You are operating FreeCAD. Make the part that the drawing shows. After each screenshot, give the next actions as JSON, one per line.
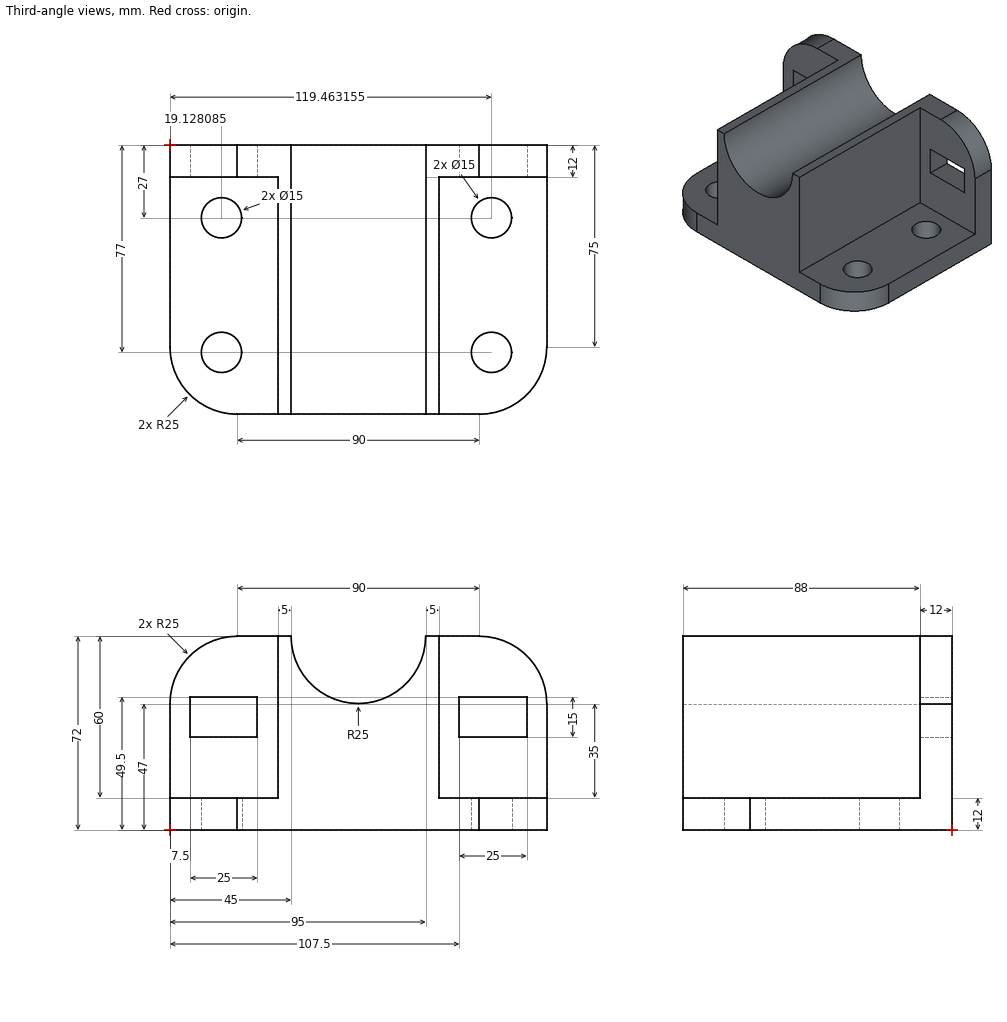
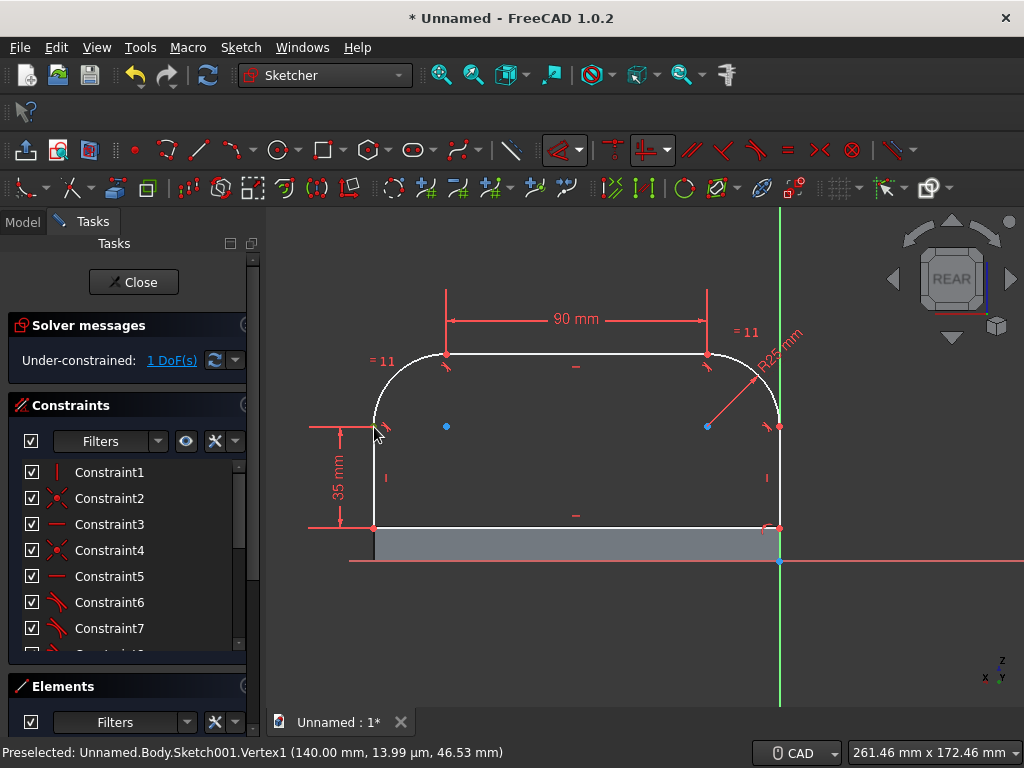
{"action": "left_click", "coordinate": [582, 150]}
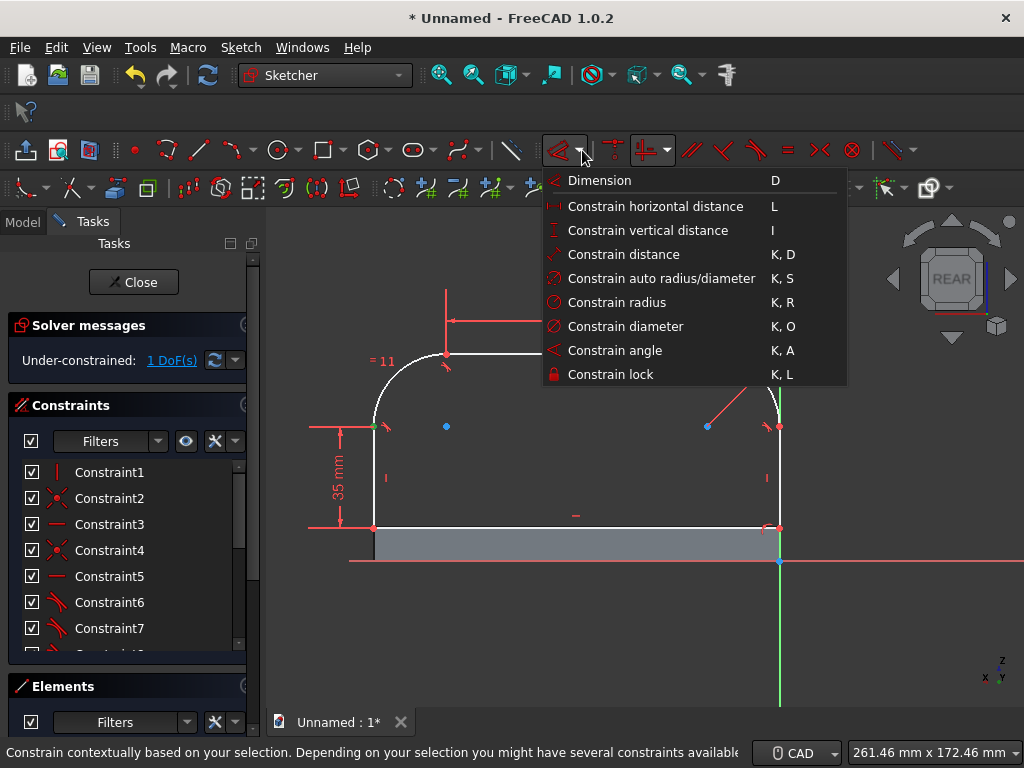
{"action": "left_click", "coordinate": [695, 230]}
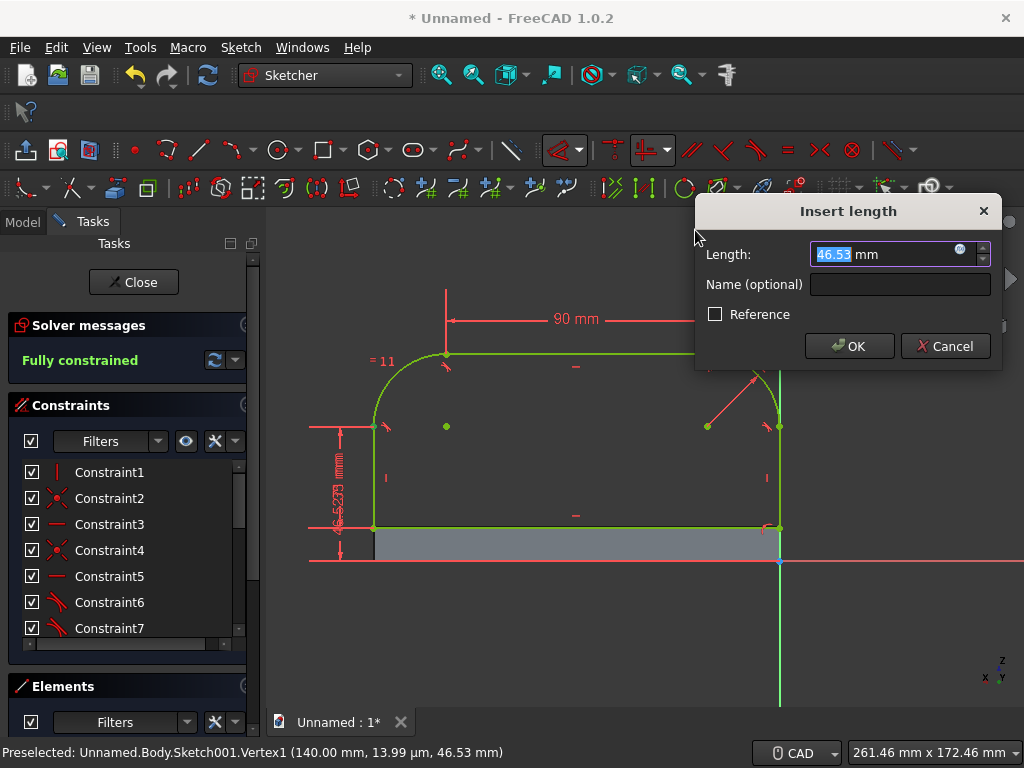
{"action": "type", "text": "47"}
{"action": "key", "text": "Return"}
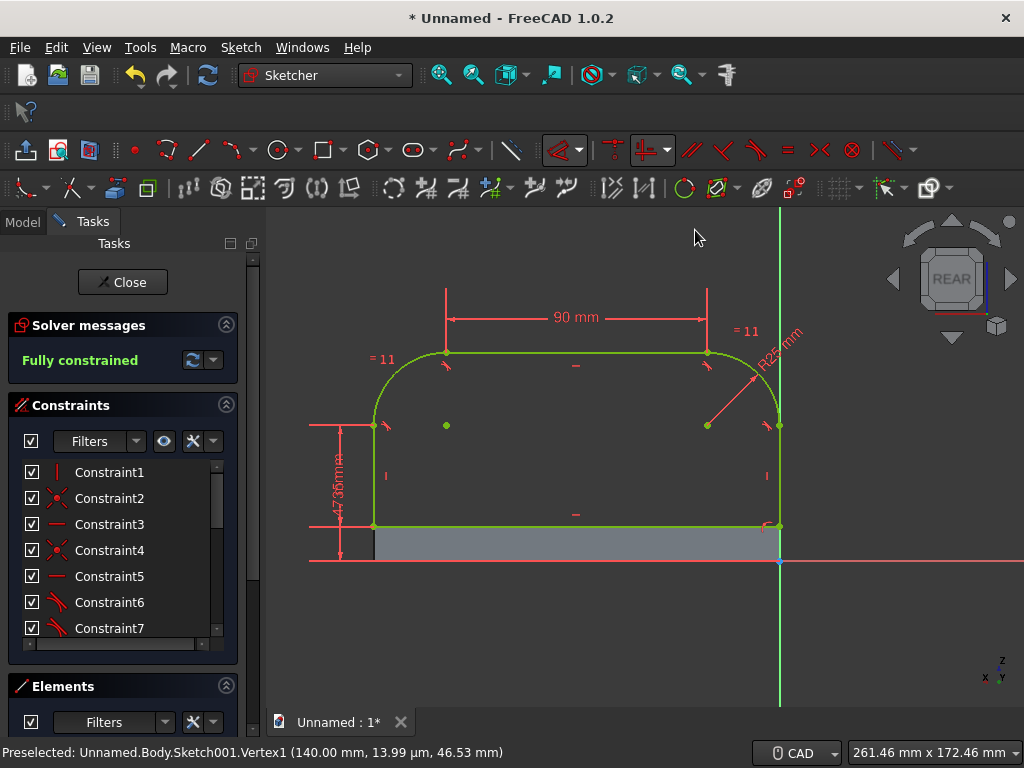
{"action": "left_click", "coordinate": [123, 282]}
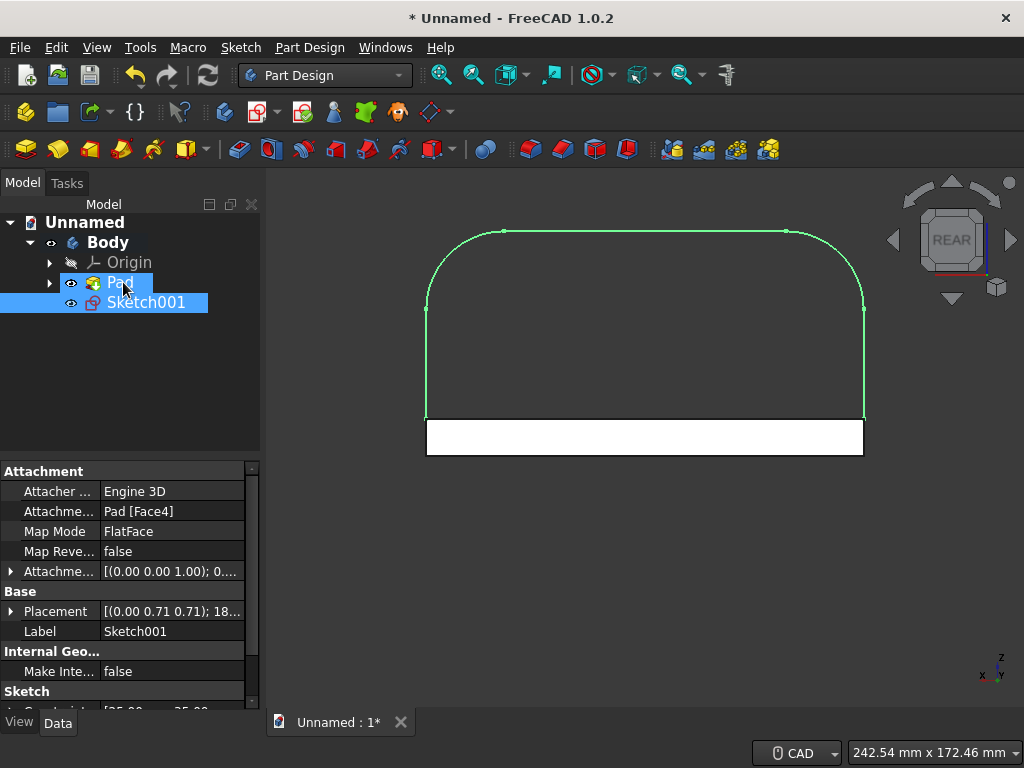
{"action": "left_click", "coordinate": [26, 150]}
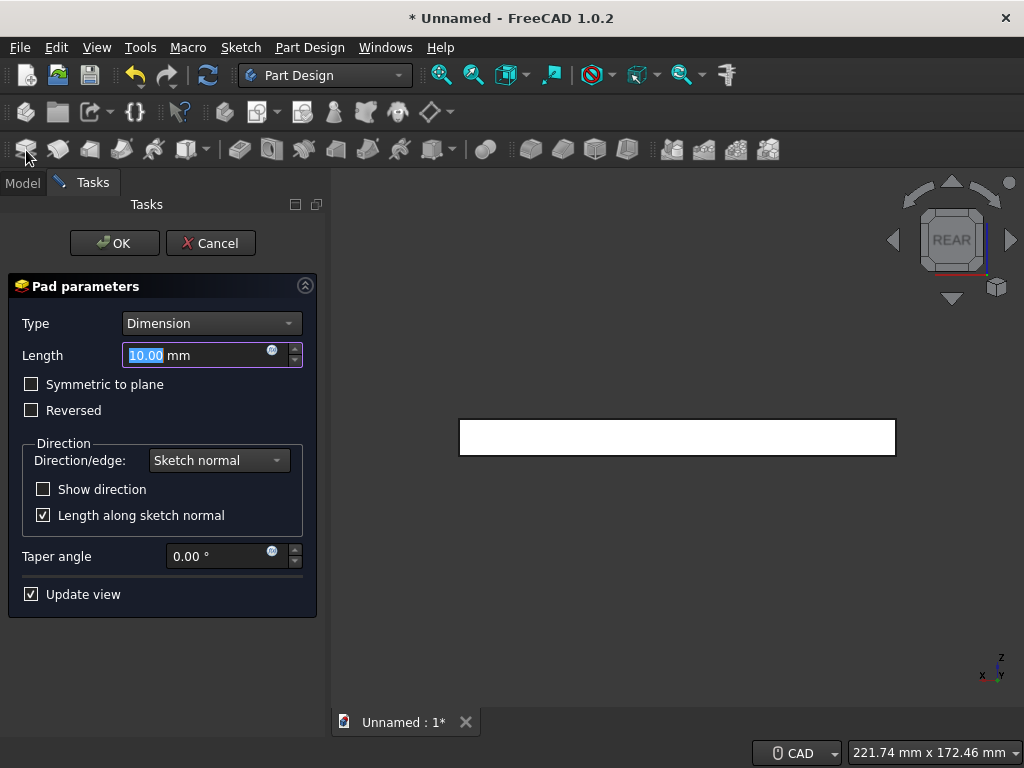
{"action": "type", "text": "12"}
{"action": "key", "text": "Tab"}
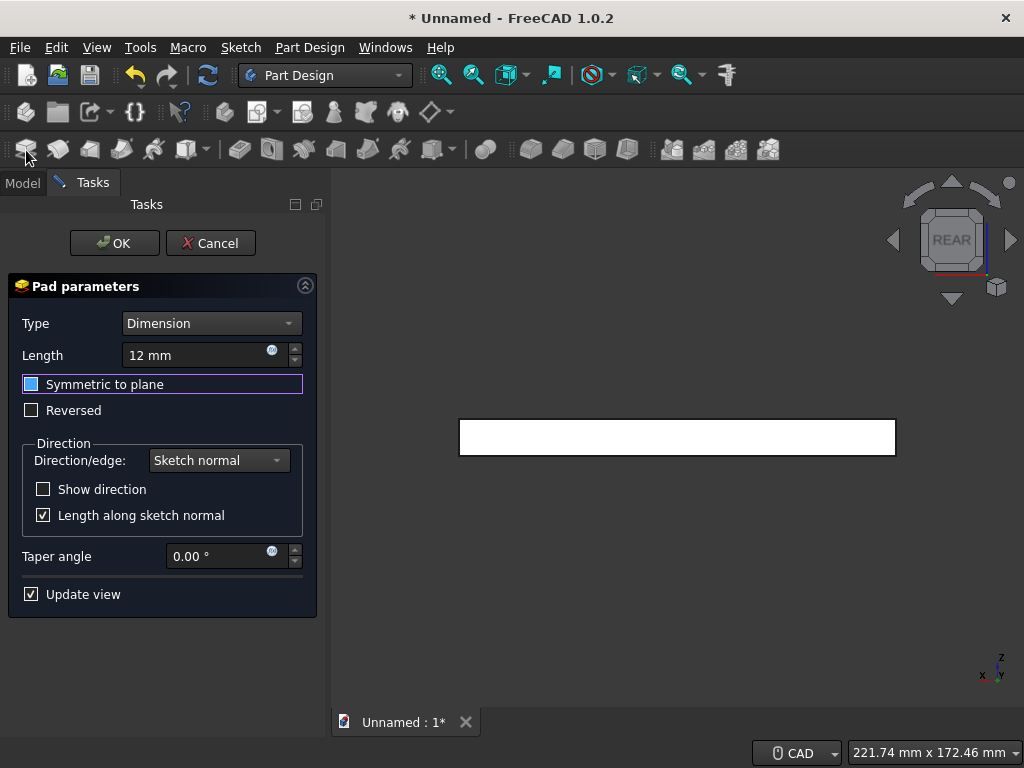
{"action": "left_click", "coordinate": [30, 410]}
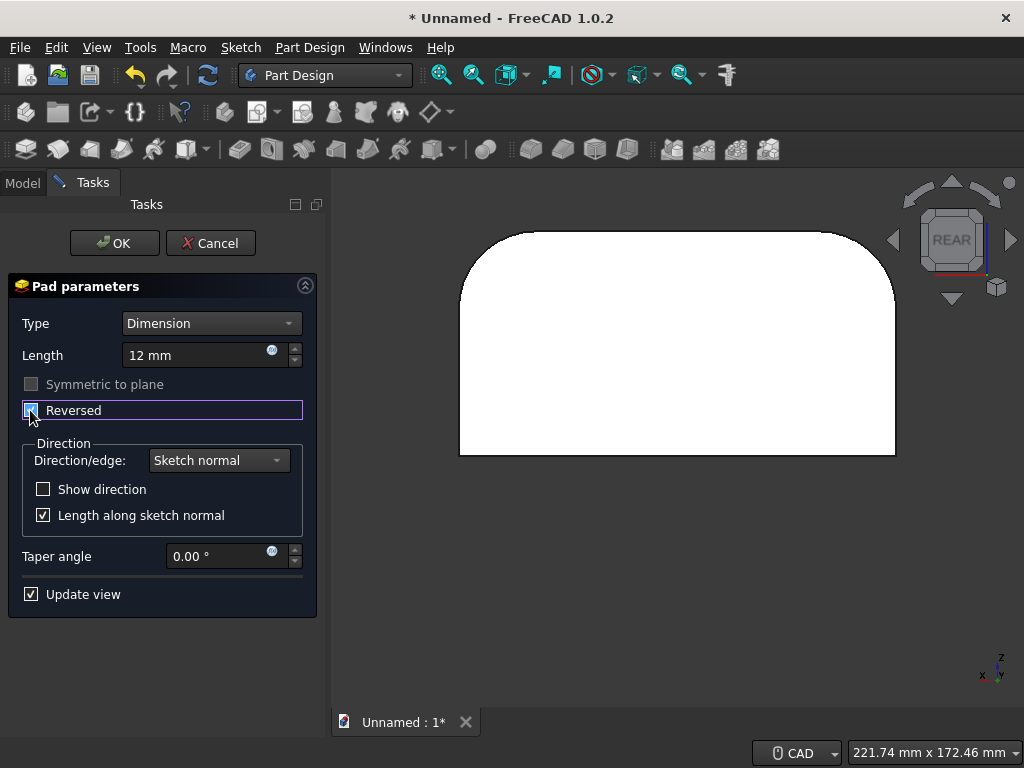
{"action": "left_click", "coordinate": [115, 243]}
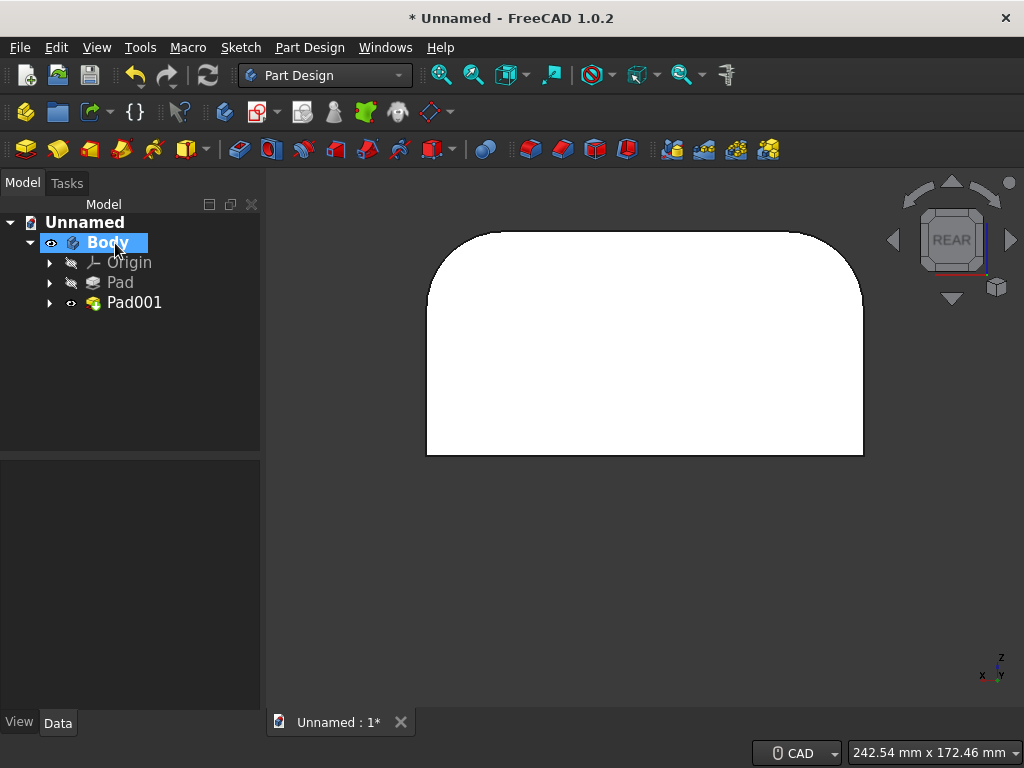
{"action": "key", "text": "0"}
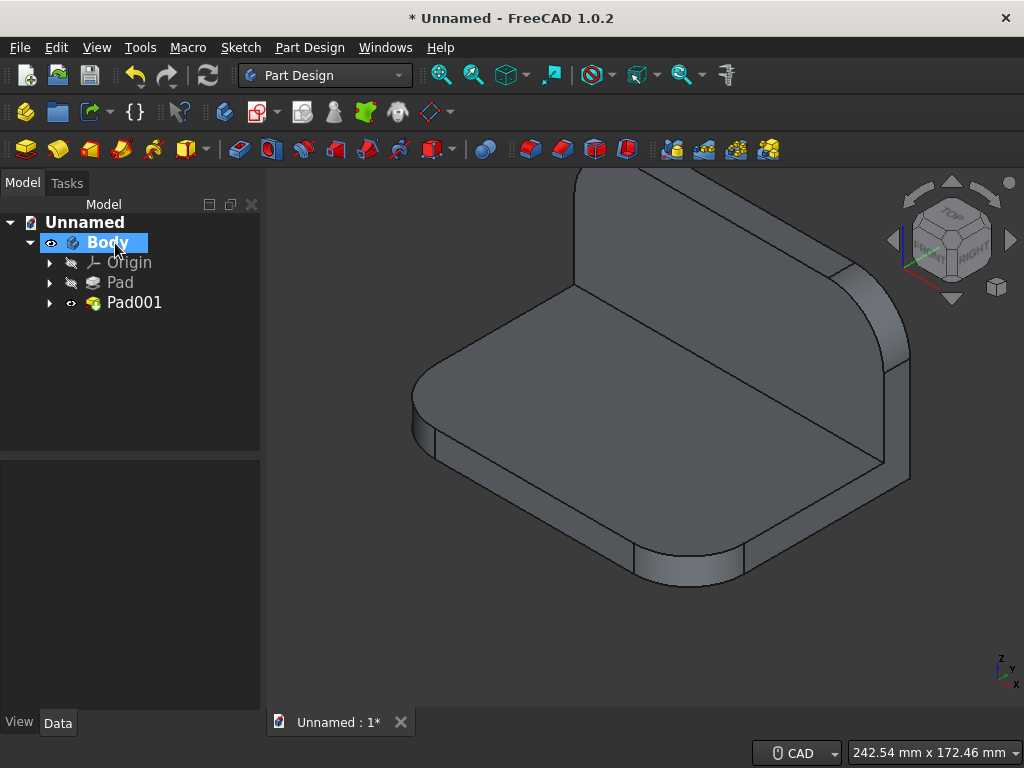
{"action": "key", "text": "v f"}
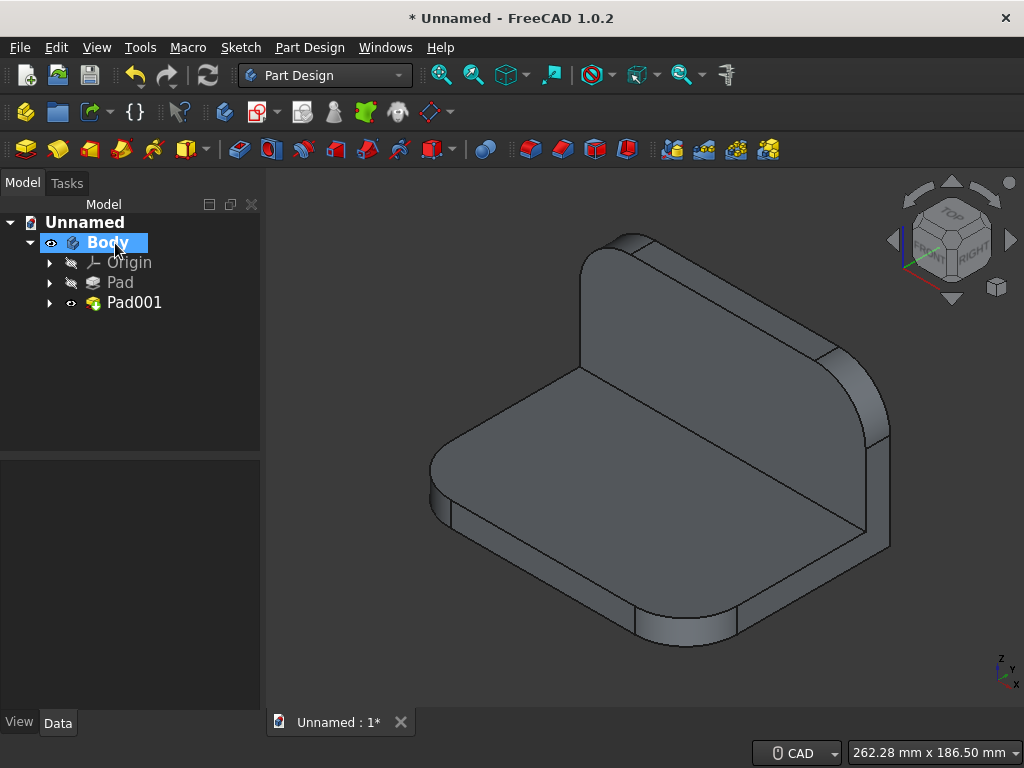
{"action": "left_click", "coordinate": [804, 425]}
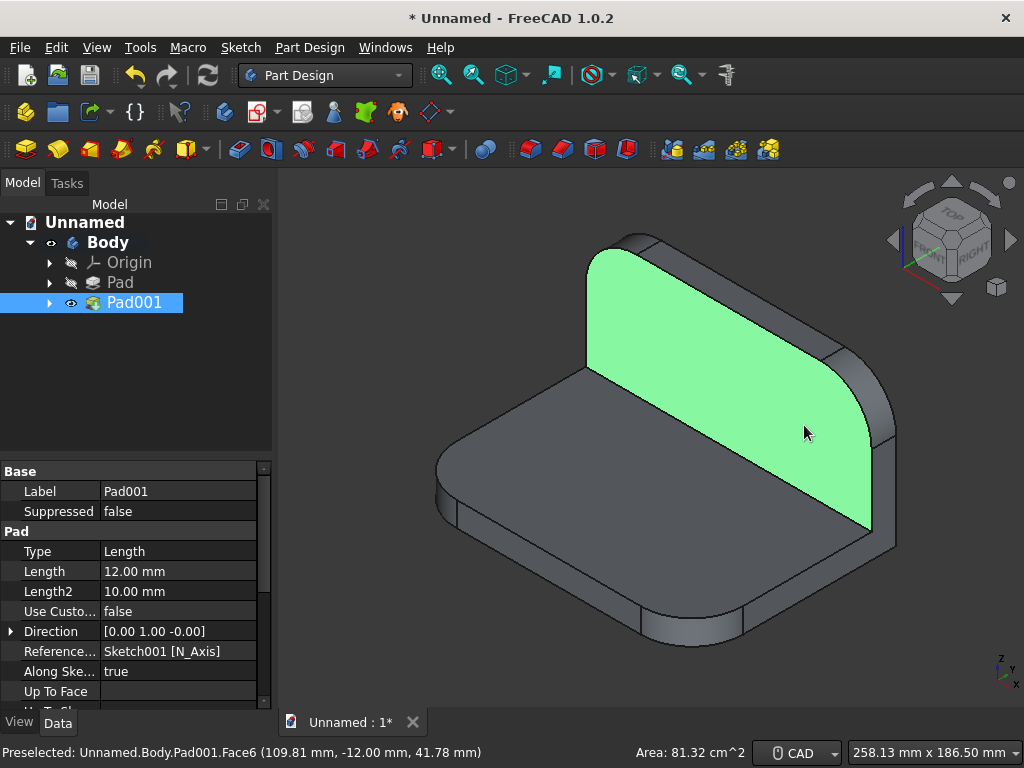
{"action": "left_click", "coordinate": [258, 112]}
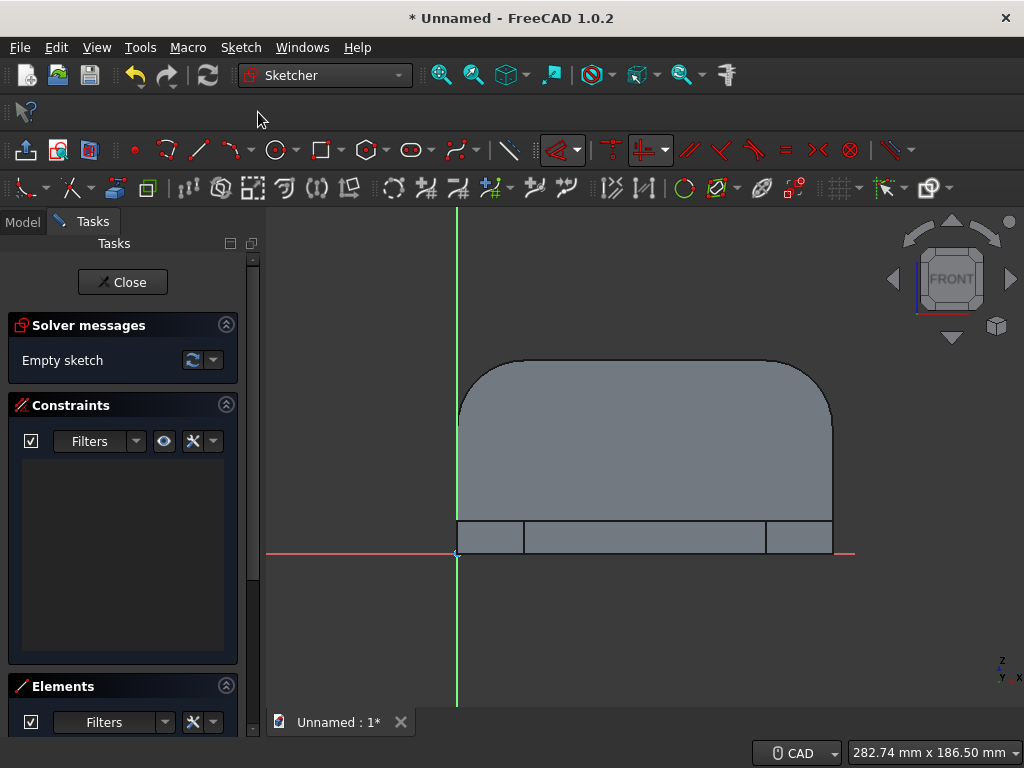
{"action": "key", "text": "q s"}